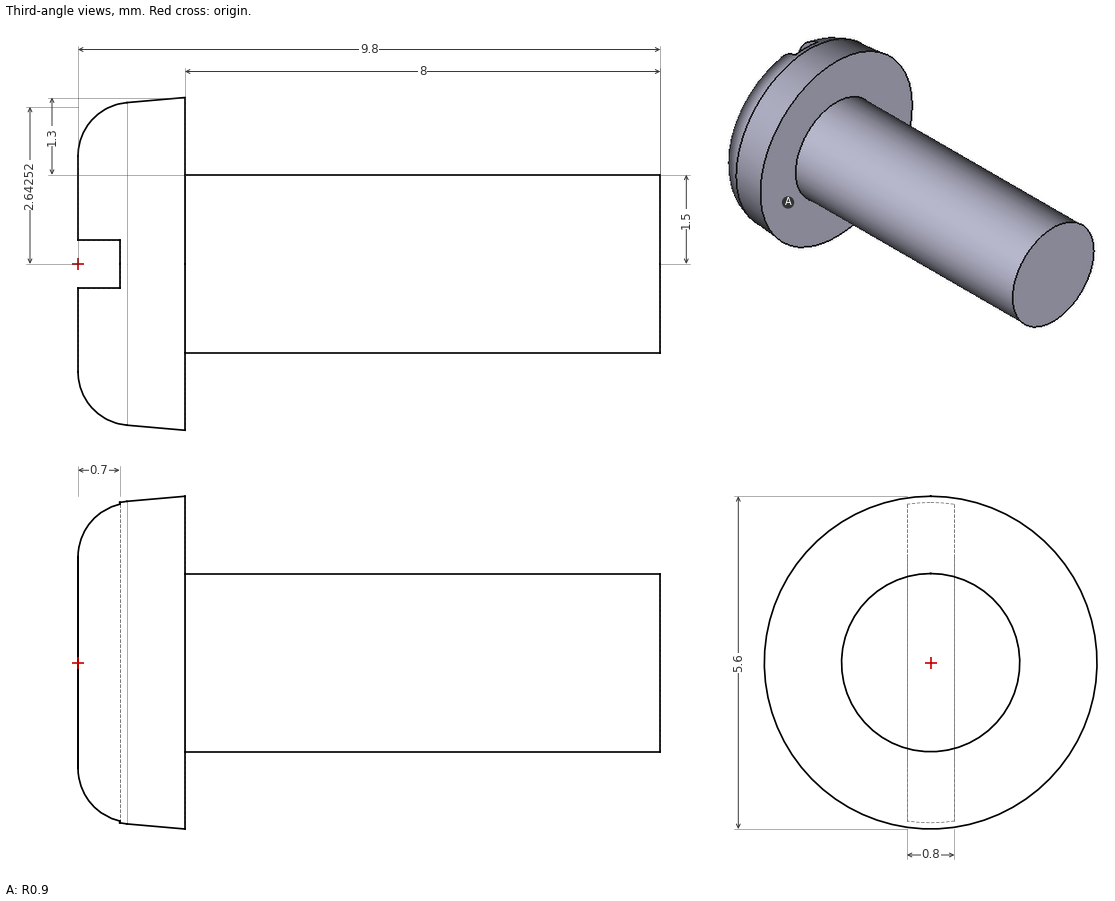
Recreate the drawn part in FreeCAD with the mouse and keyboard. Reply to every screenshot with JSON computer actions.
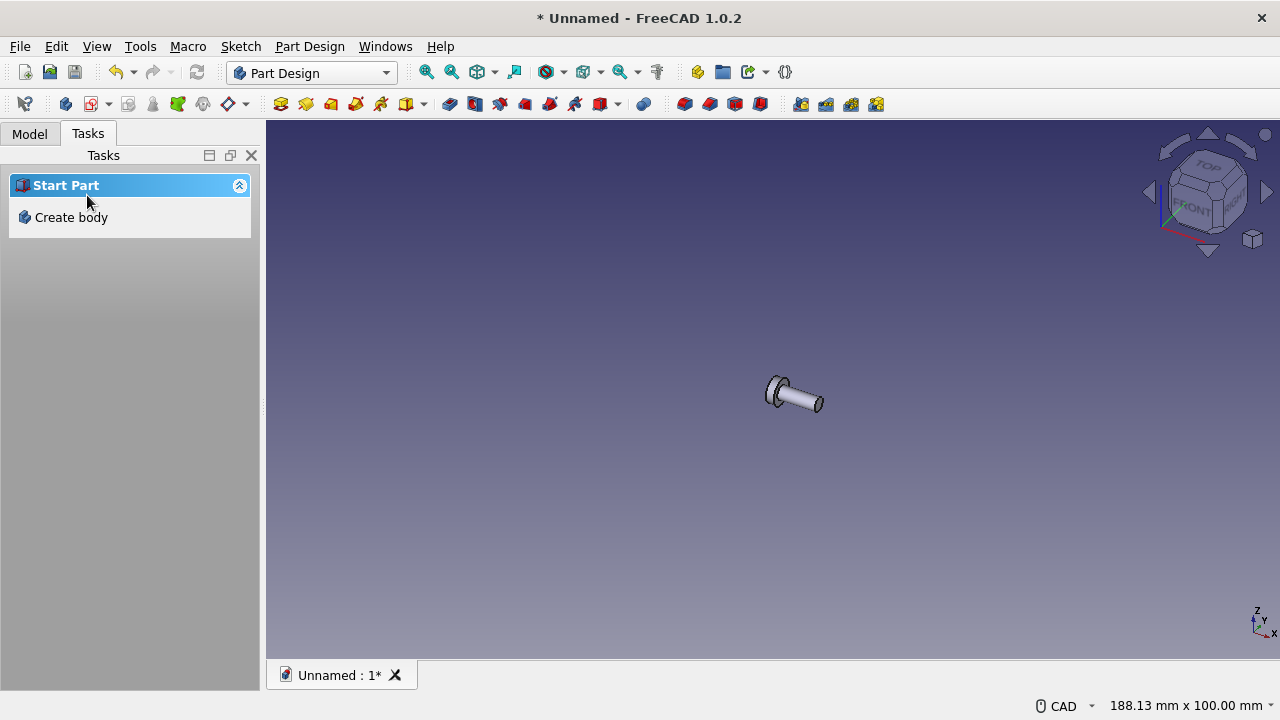
{"action": "left_click", "coordinate": [427, 72]}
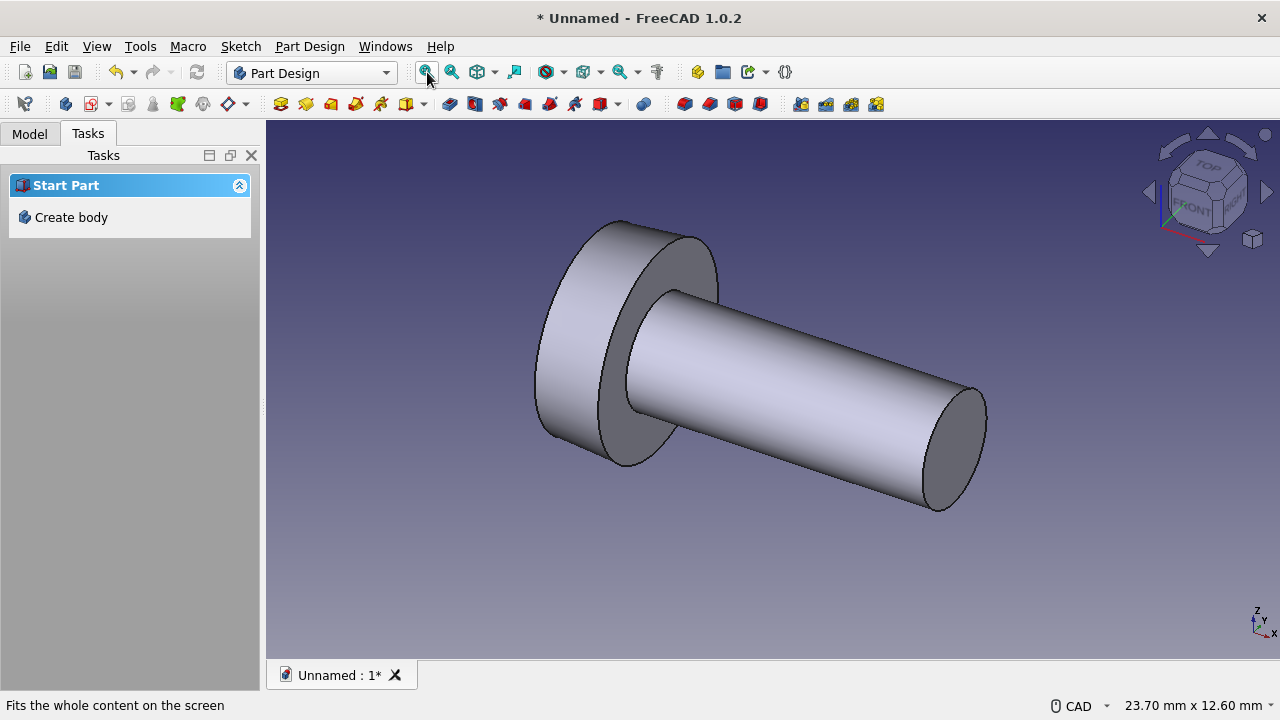
{"action": "key", "text": "0"}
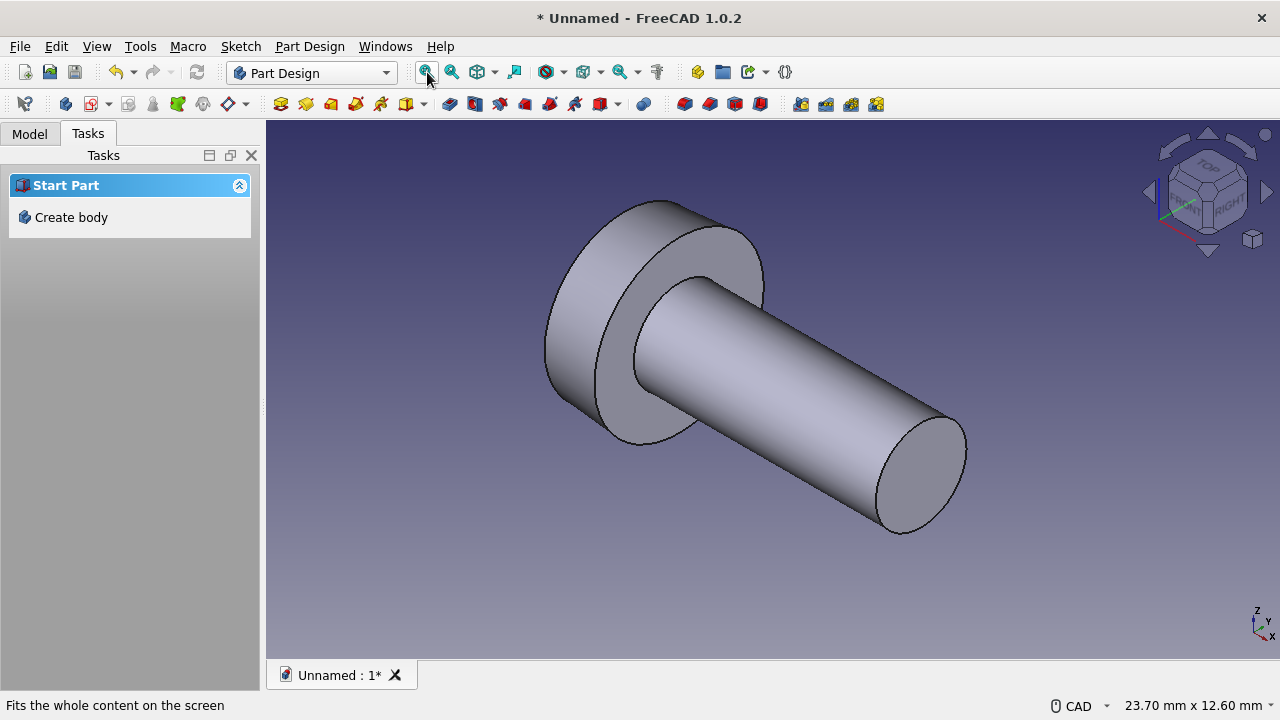
{"action": "key", "text": "2"}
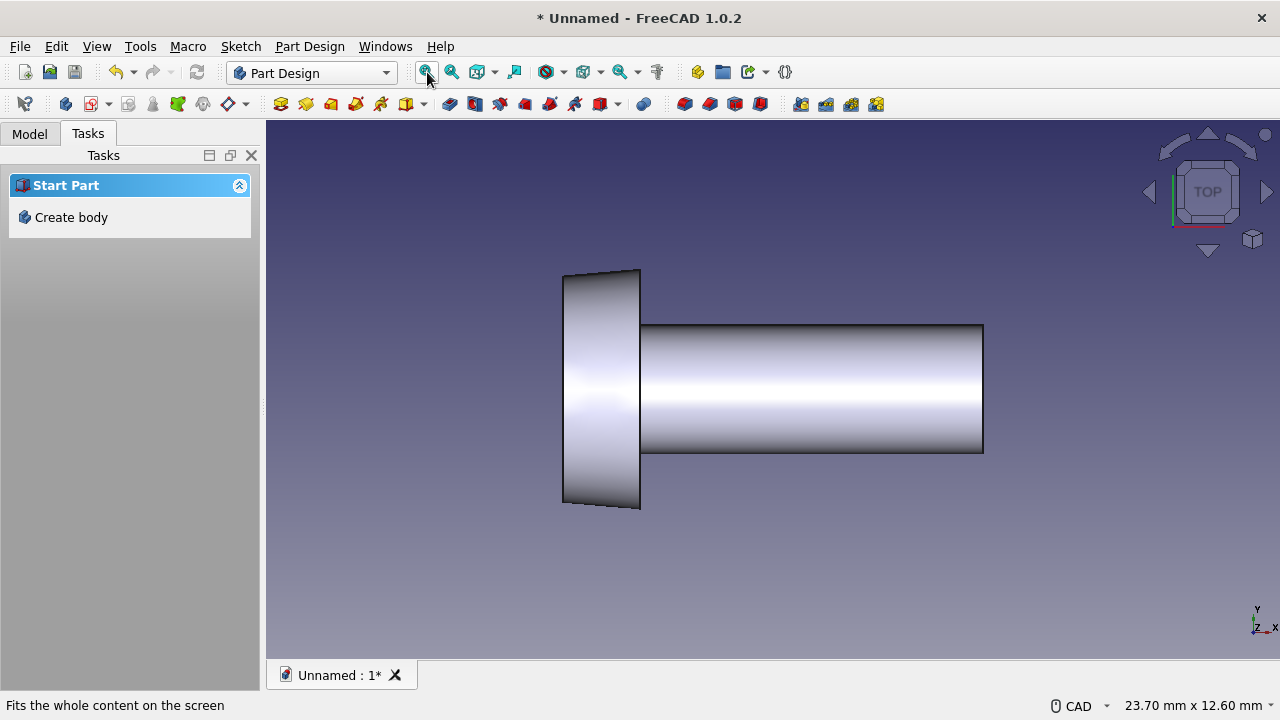
{"action": "key", "text": "v f"}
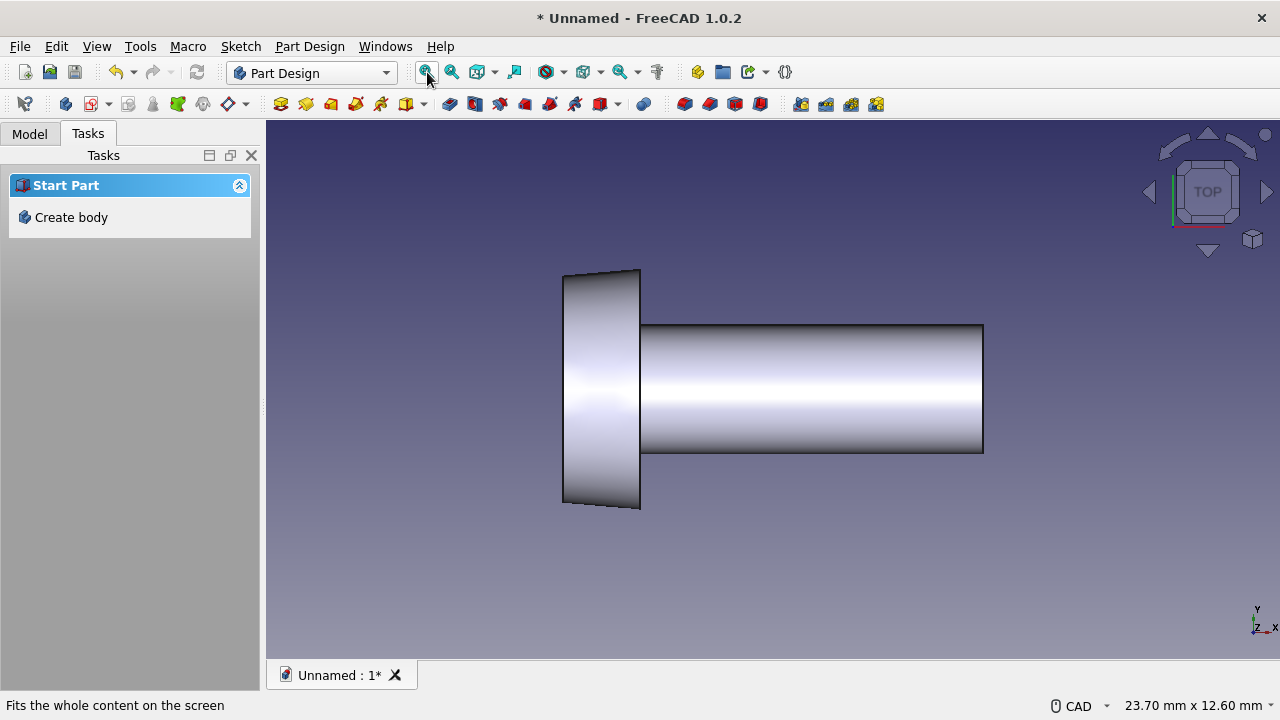
{"action": "left_click", "coordinate": [563, 424]}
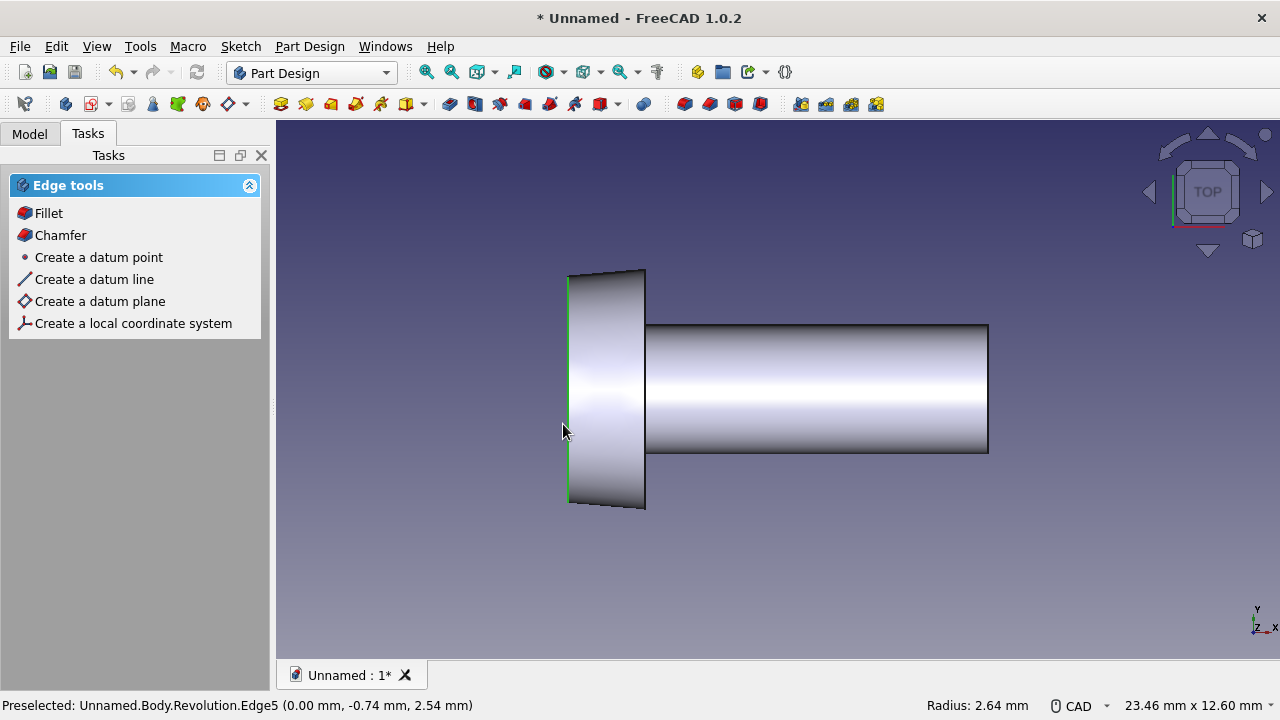
{"action": "left_click", "coordinate": [685, 104]}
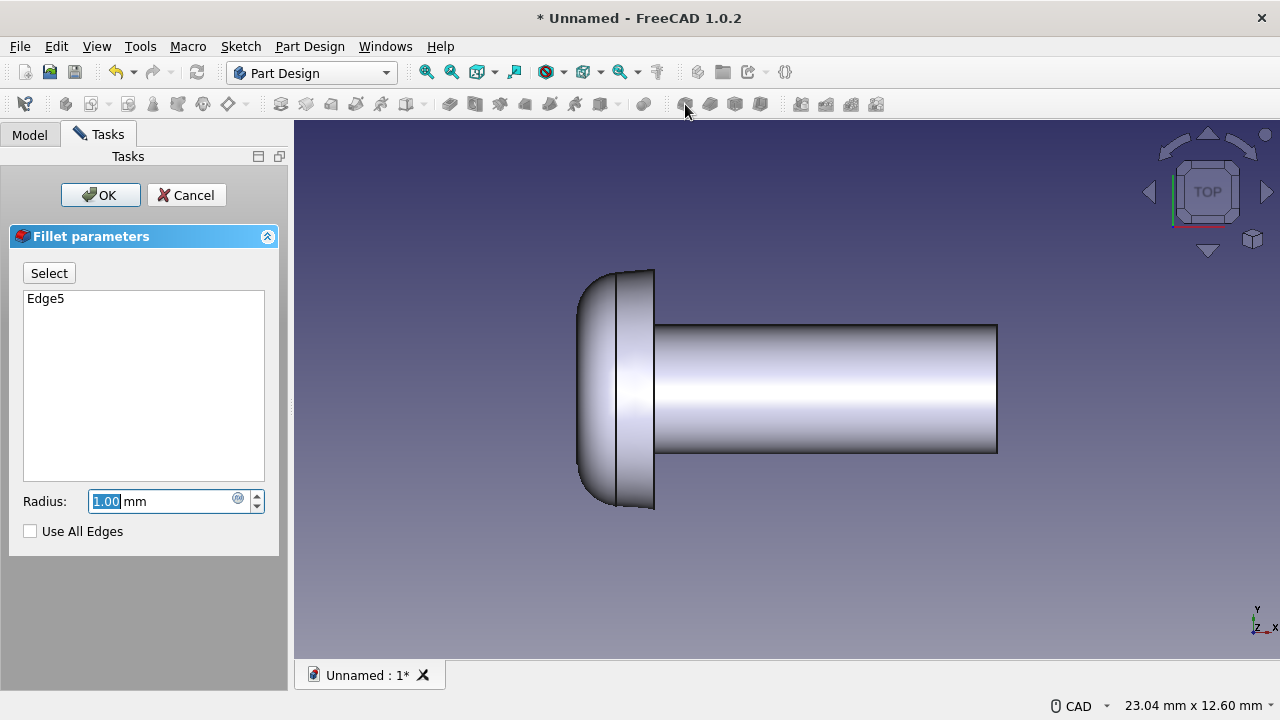
{"action": "type", "text": "0.9"}
{"action": "key", "text": "Tab"}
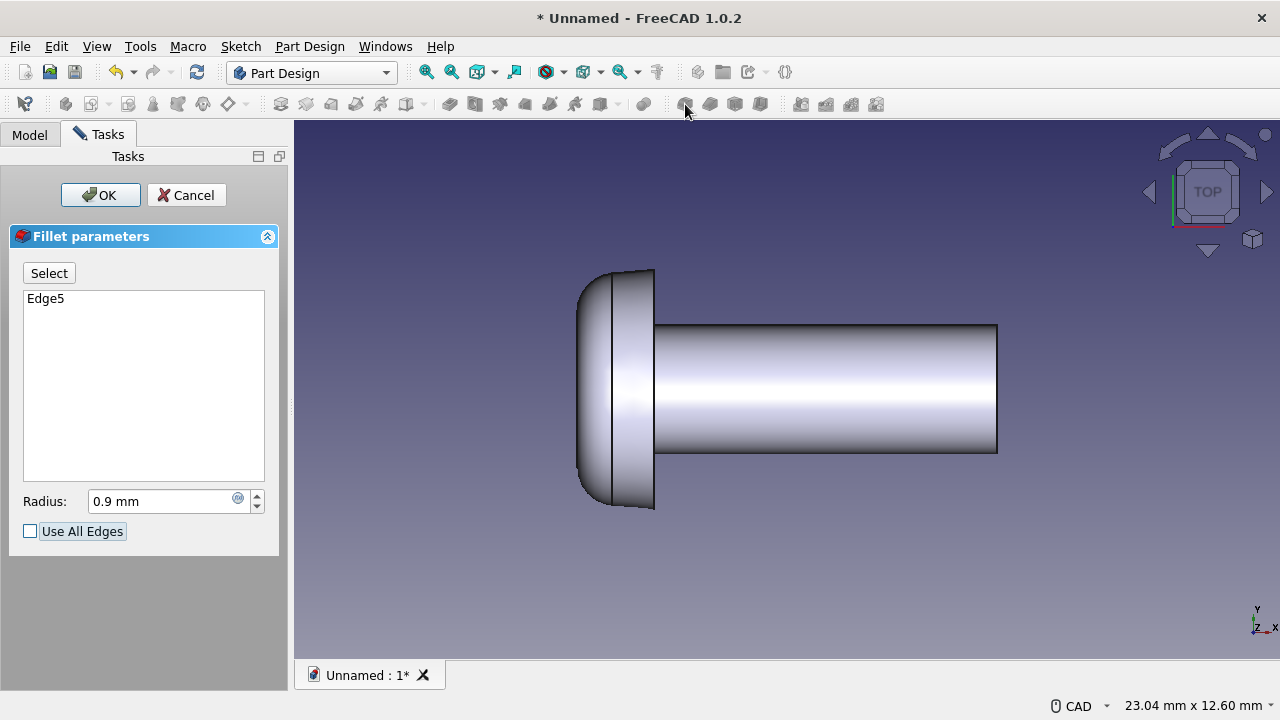
{"action": "left_click", "coordinate": [101, 195]}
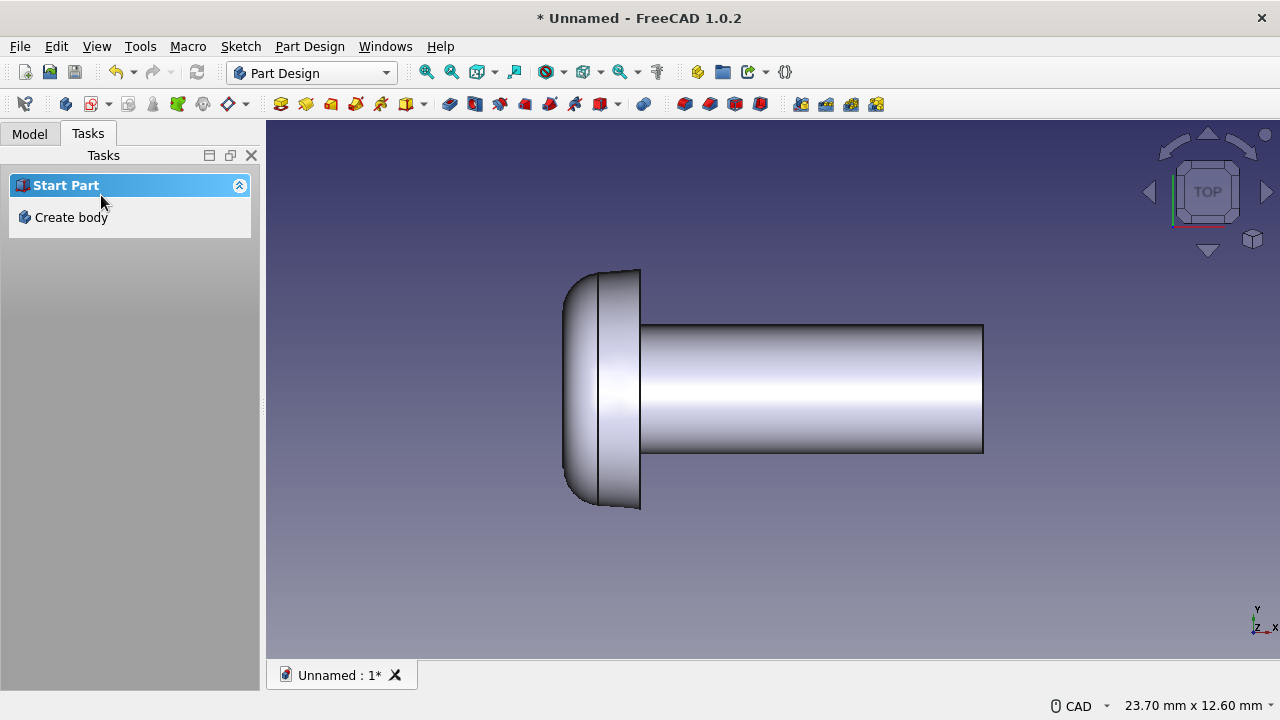
{"action": "left_click", "coordinate": [427, 72]}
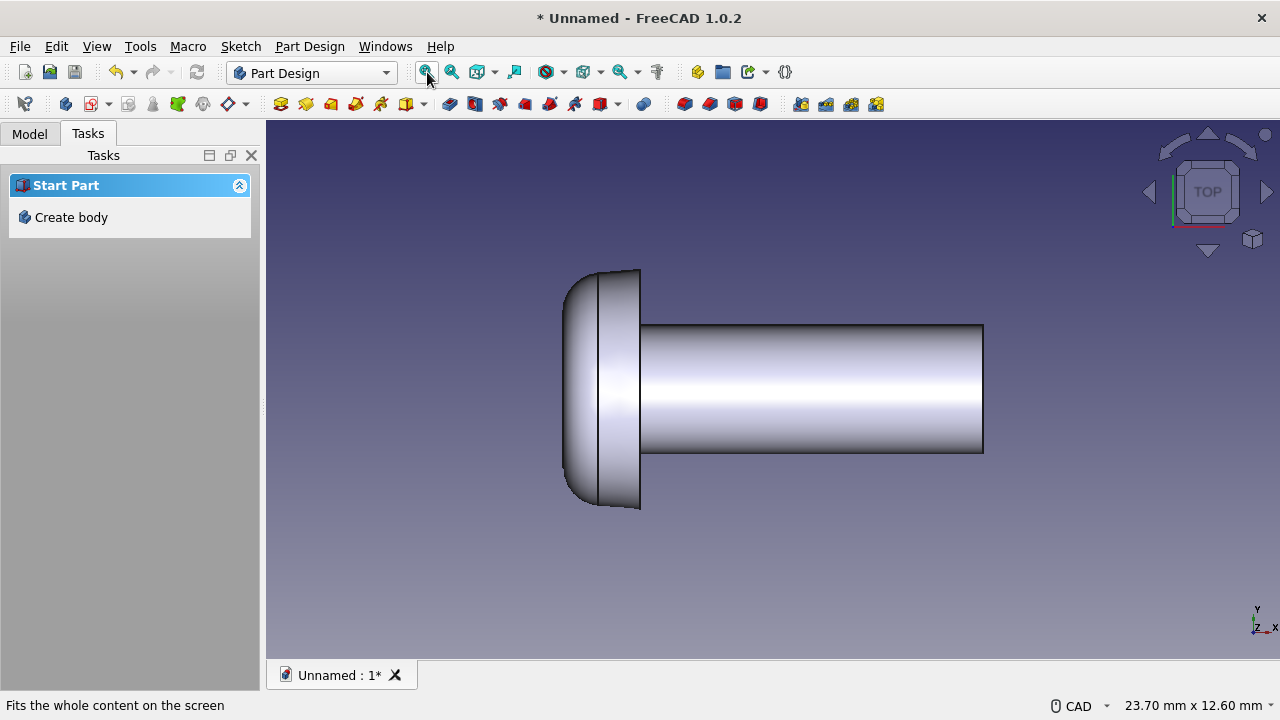
{"action": "key", "text": "6"}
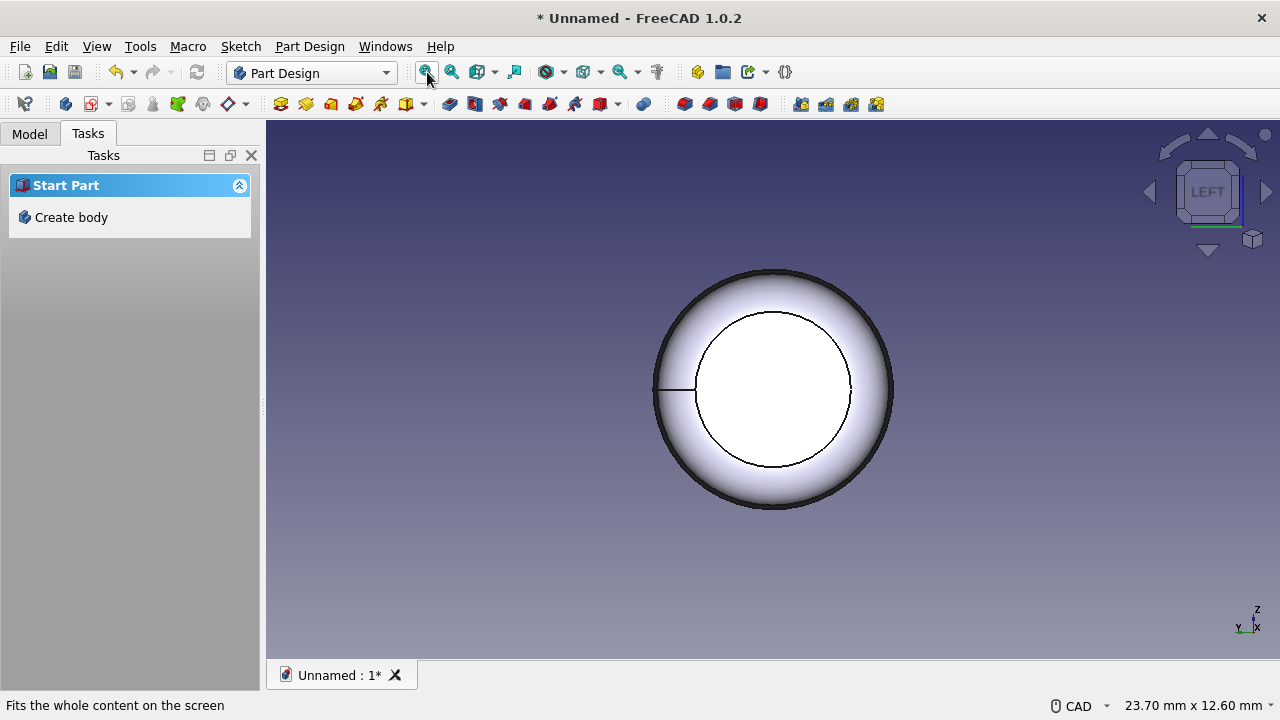
{"action": "left_click", "coordinate": [427, 72]}